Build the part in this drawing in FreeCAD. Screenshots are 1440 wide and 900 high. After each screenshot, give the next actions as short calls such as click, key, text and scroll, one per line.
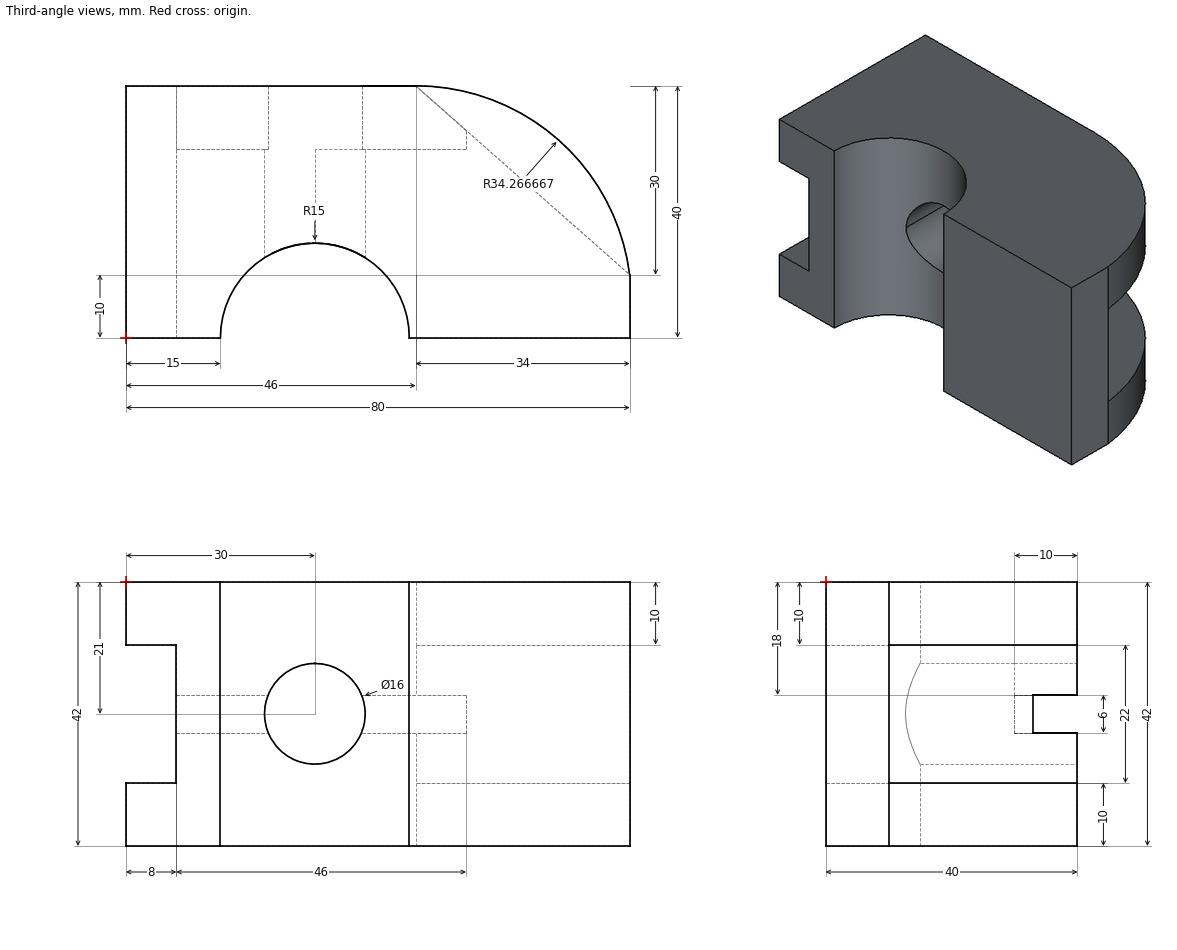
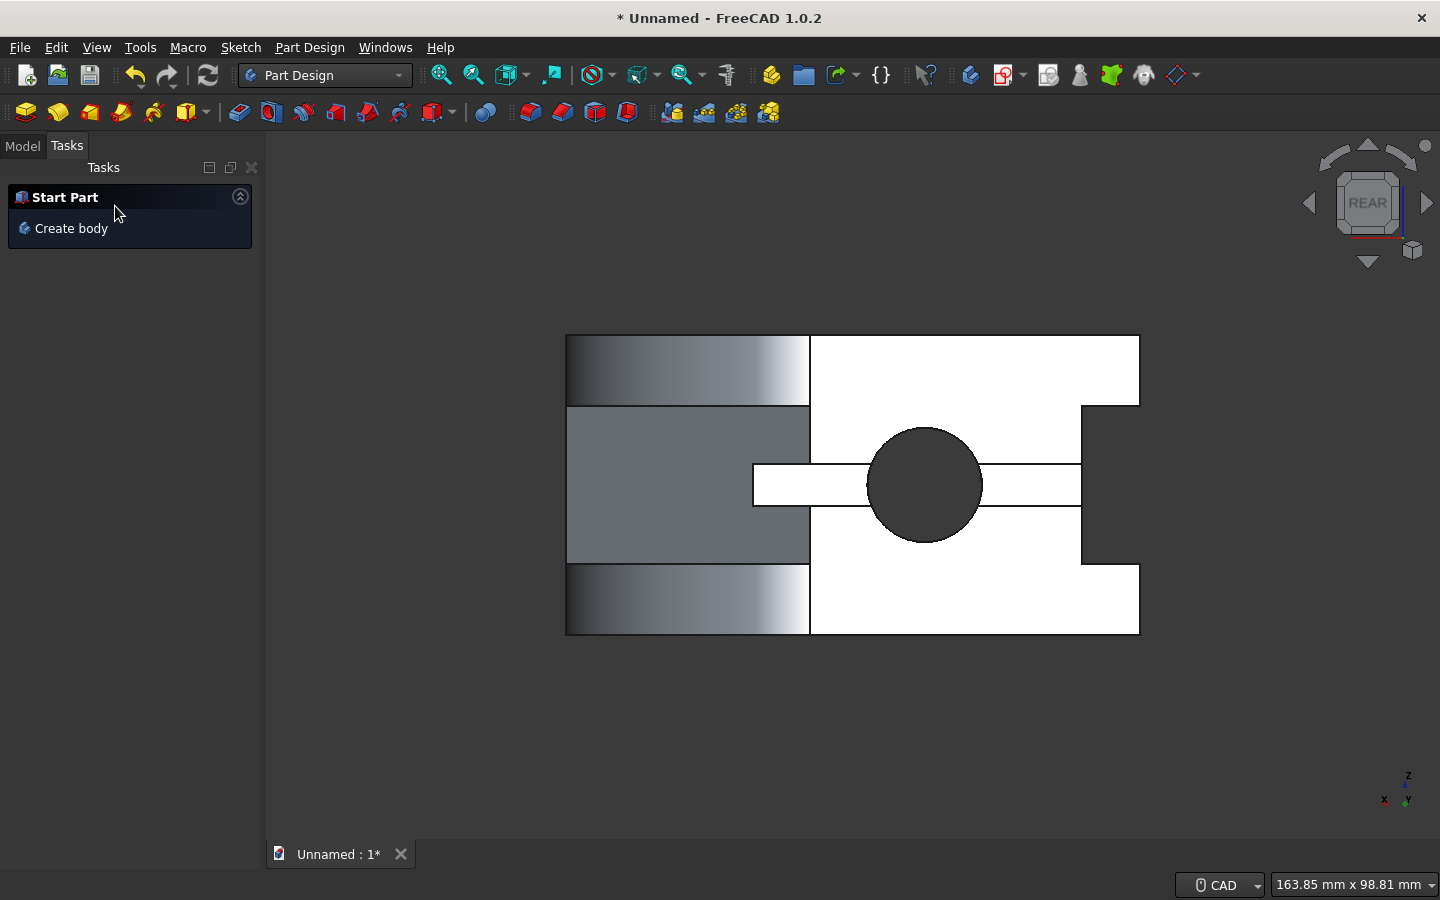
key(0)